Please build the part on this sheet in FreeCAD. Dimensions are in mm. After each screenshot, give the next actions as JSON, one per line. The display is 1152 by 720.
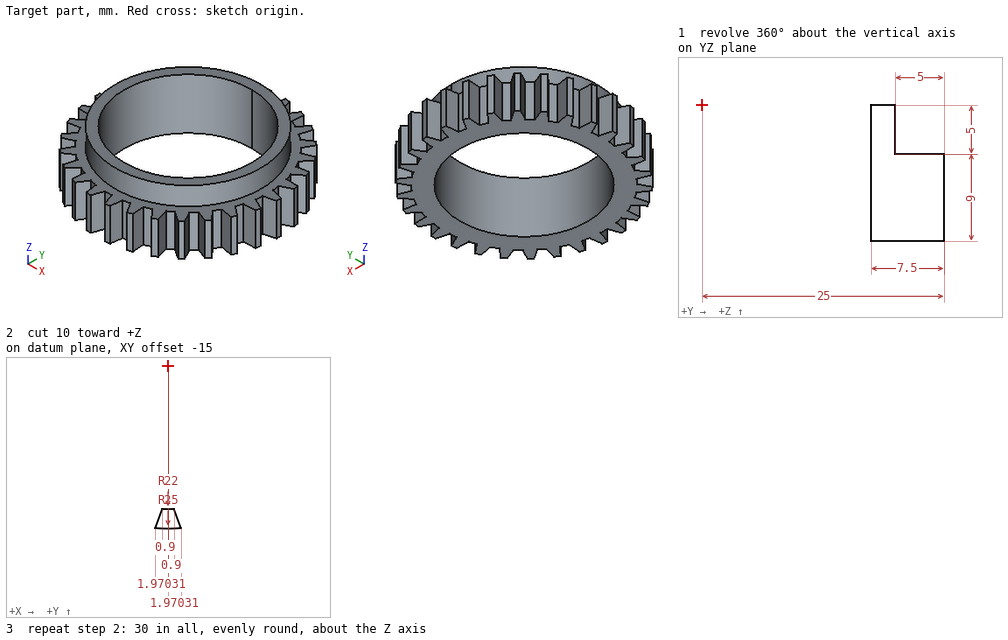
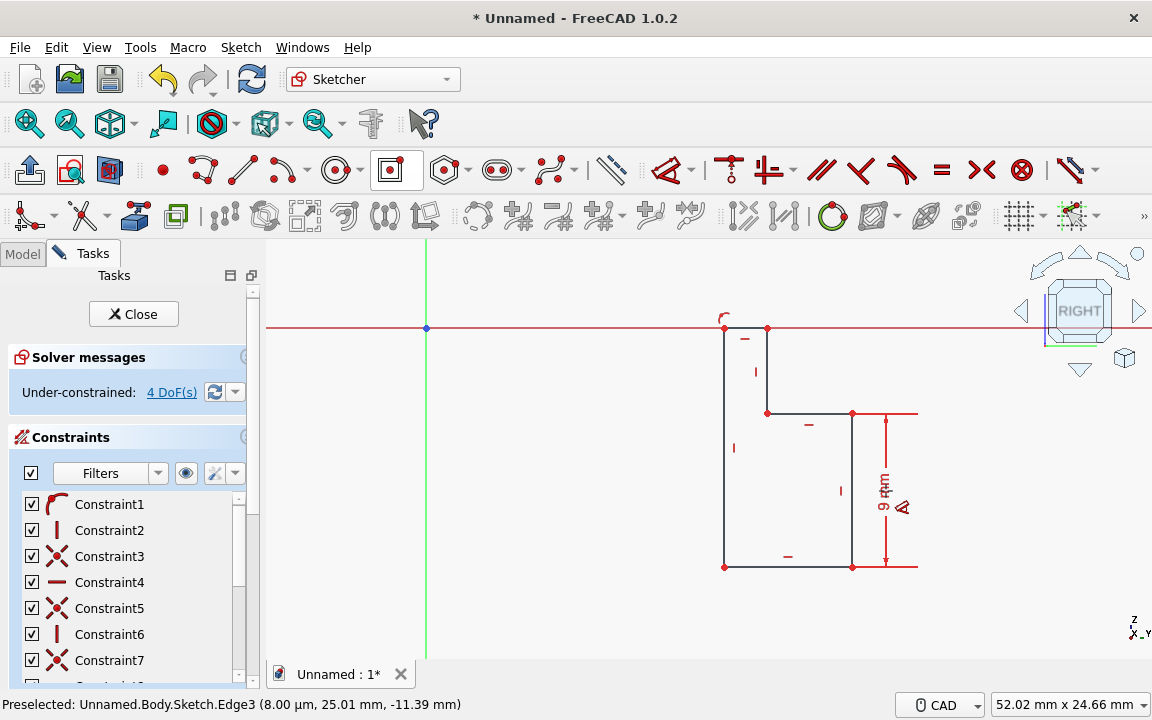
{"action": "left_click", "coordinate": [826, 414]}
{"action": "left_click", "coordinate": [809, 380]}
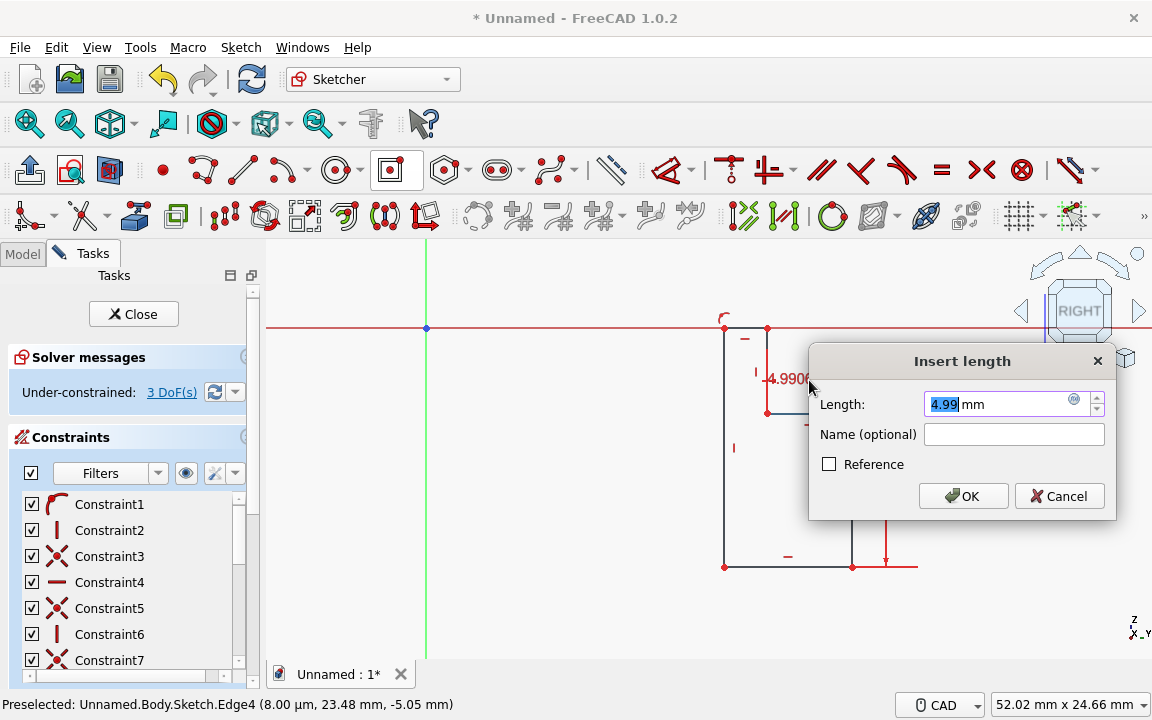
{"action": "type", "text": "5"}
{"action": "key", "text": "Return"}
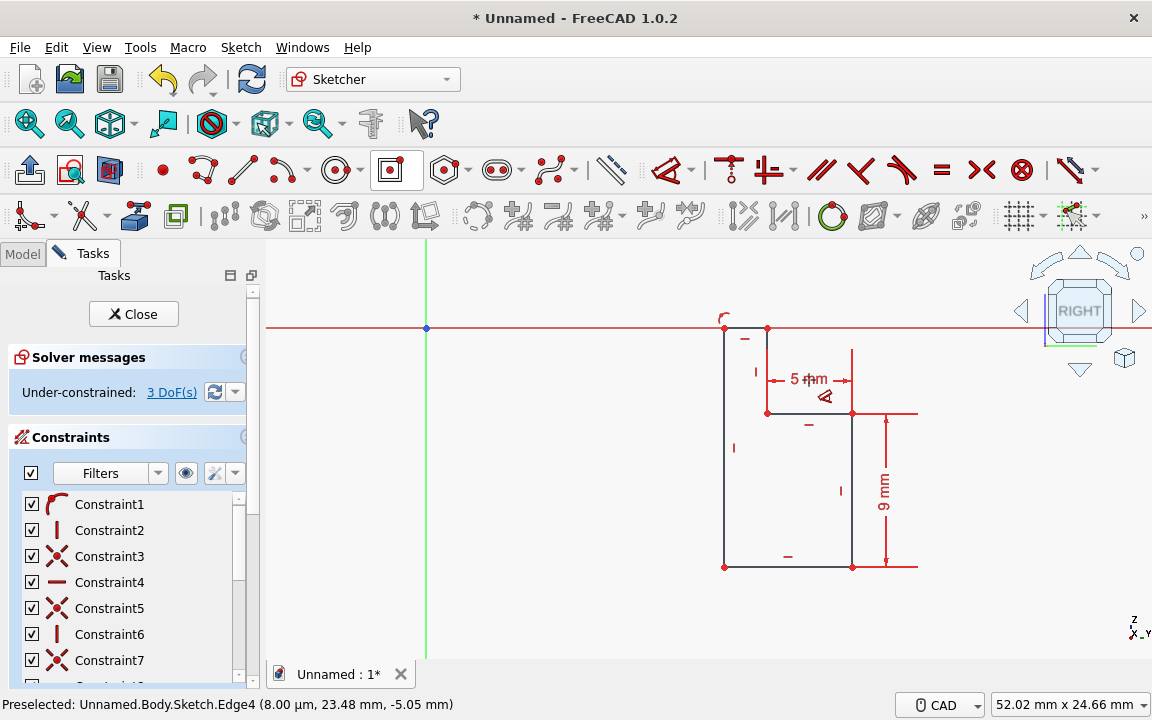
{"action": "left_click", "coordinate": [767, 388]}
{"action": "left_click", "coordinate": [801, 351]}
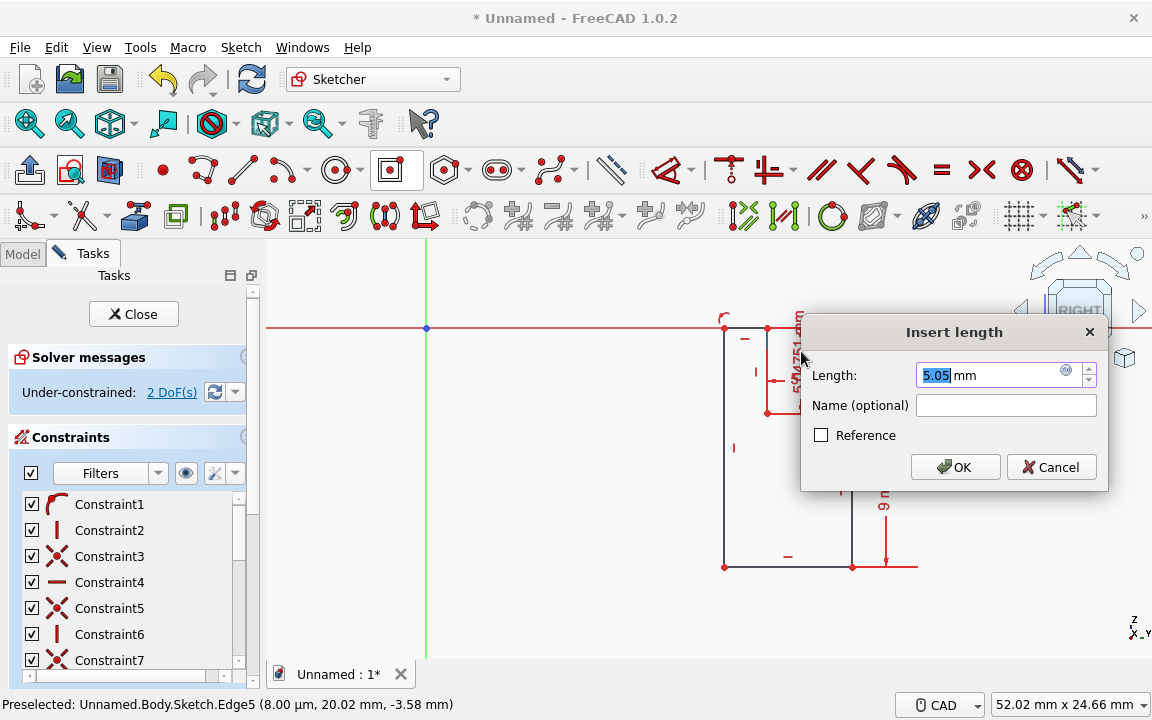
{"action": "type", "text": "5"}
{"action": "key", "text": "Return"}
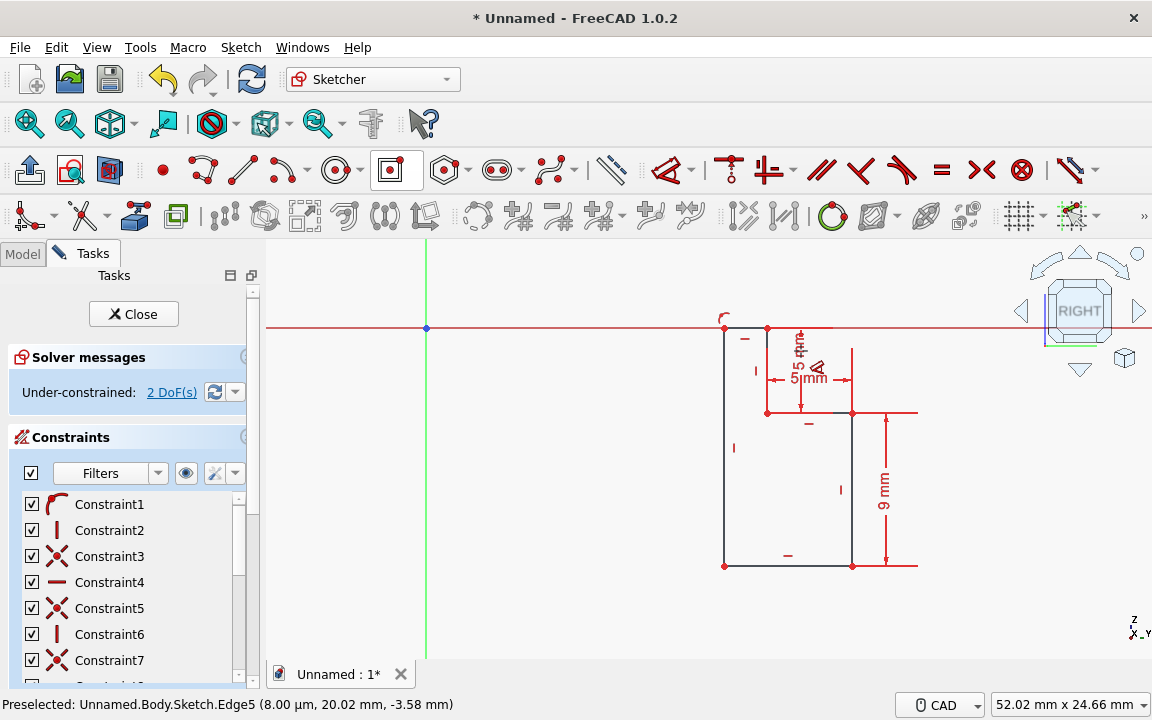
{"action": "left_click", "coordinate": [762, 566]}
{"action": "left_click", "coordinate": [788, 600]}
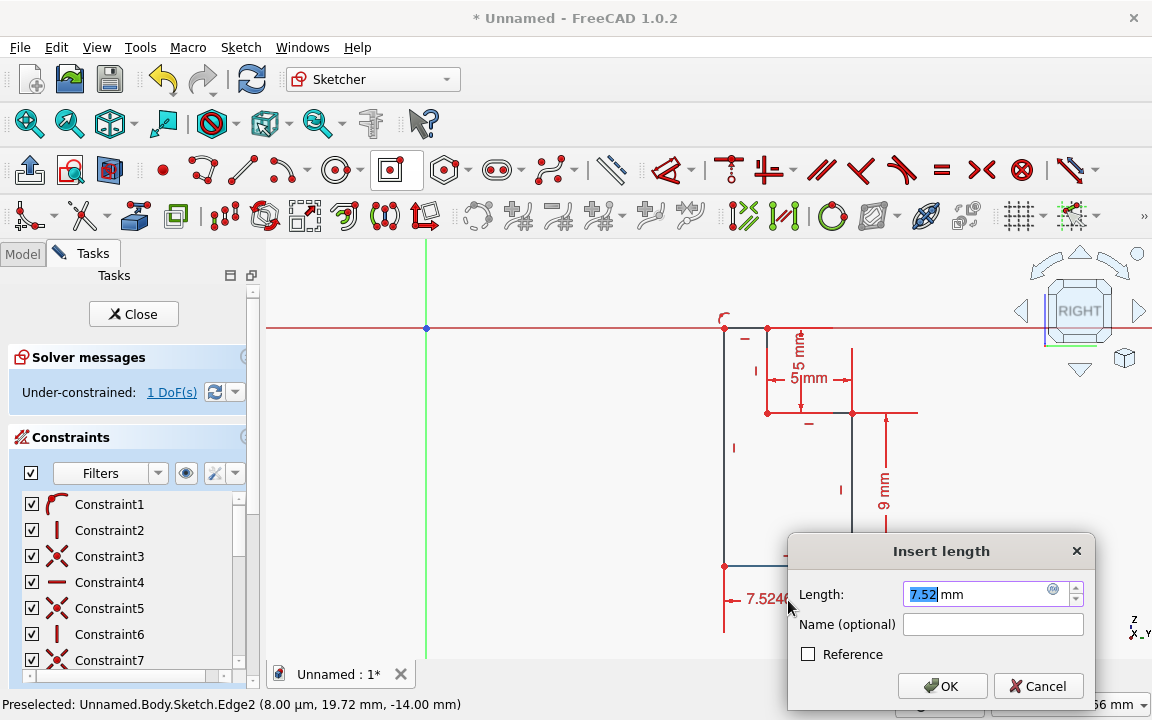
{"action": "type", "text": "7.5"}
{"action": "key", "text": "Return"}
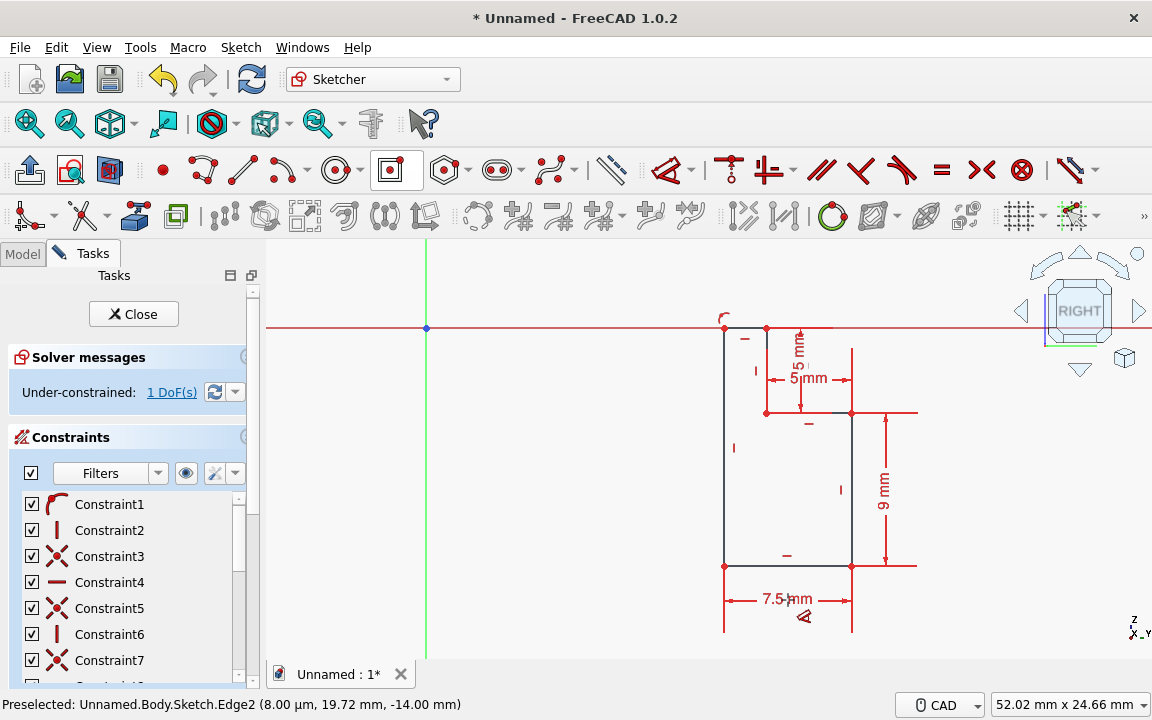
{"action": "left_click", "coordinate": [852, 566]}
{"action": "left_click", "coordinate": [639, 600]}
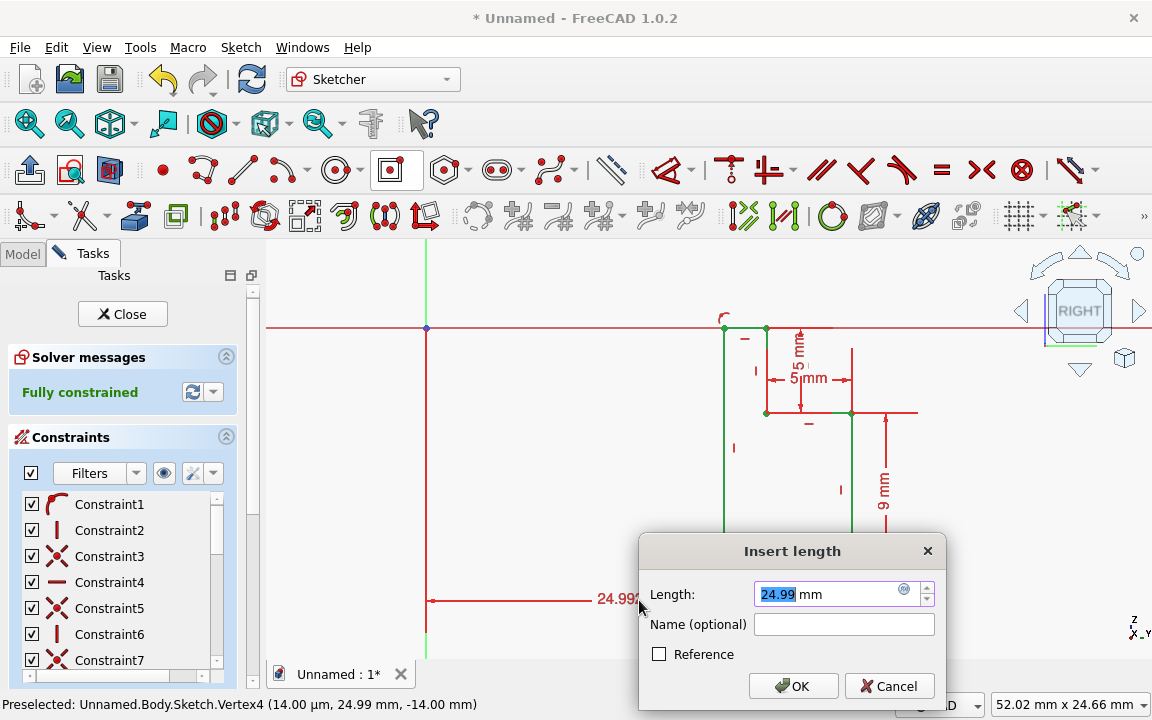
{"action": "type", "text": "25"}
{"action": "key", "text": "Return"}
{"action": "key", "text": "Escape"}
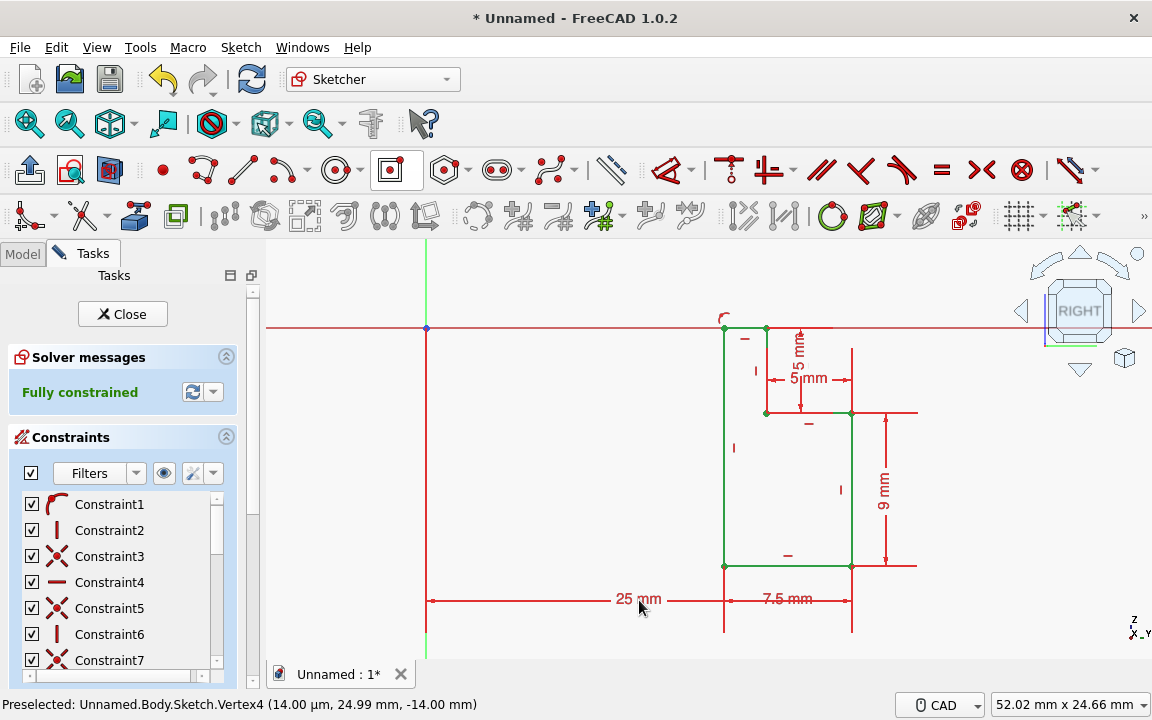
{"action": "left_click", "coordinate": [123, 314]}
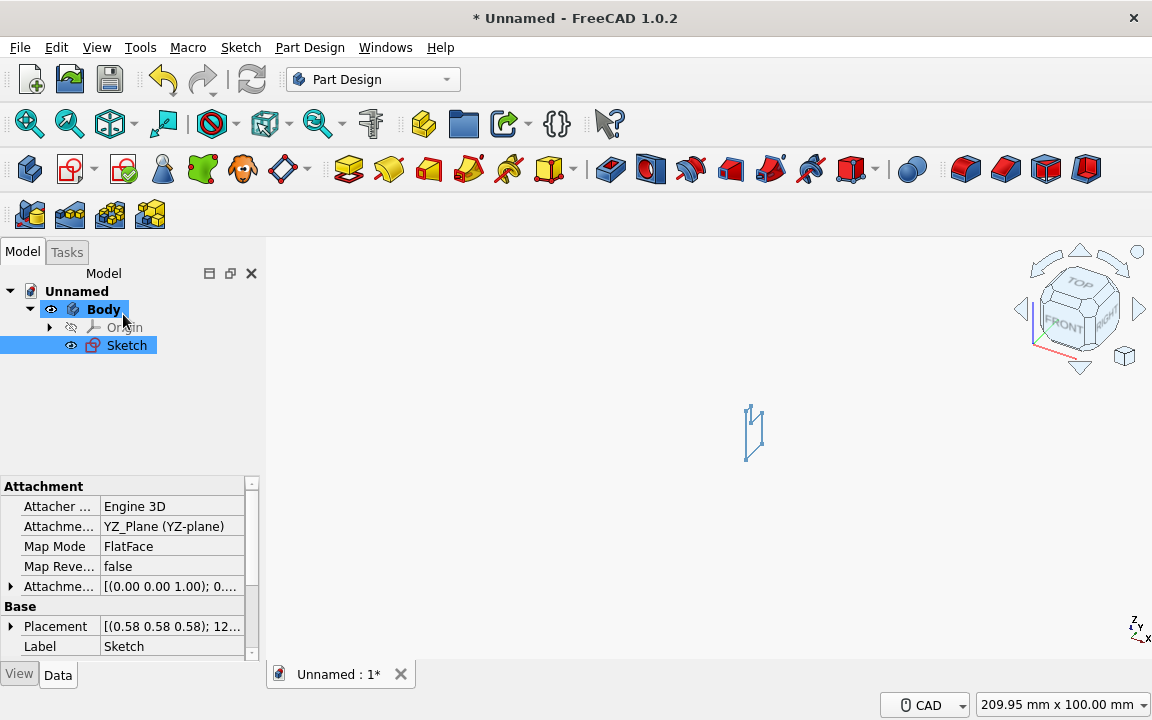
{"action": "left_click", "coordinate": [390, 170]}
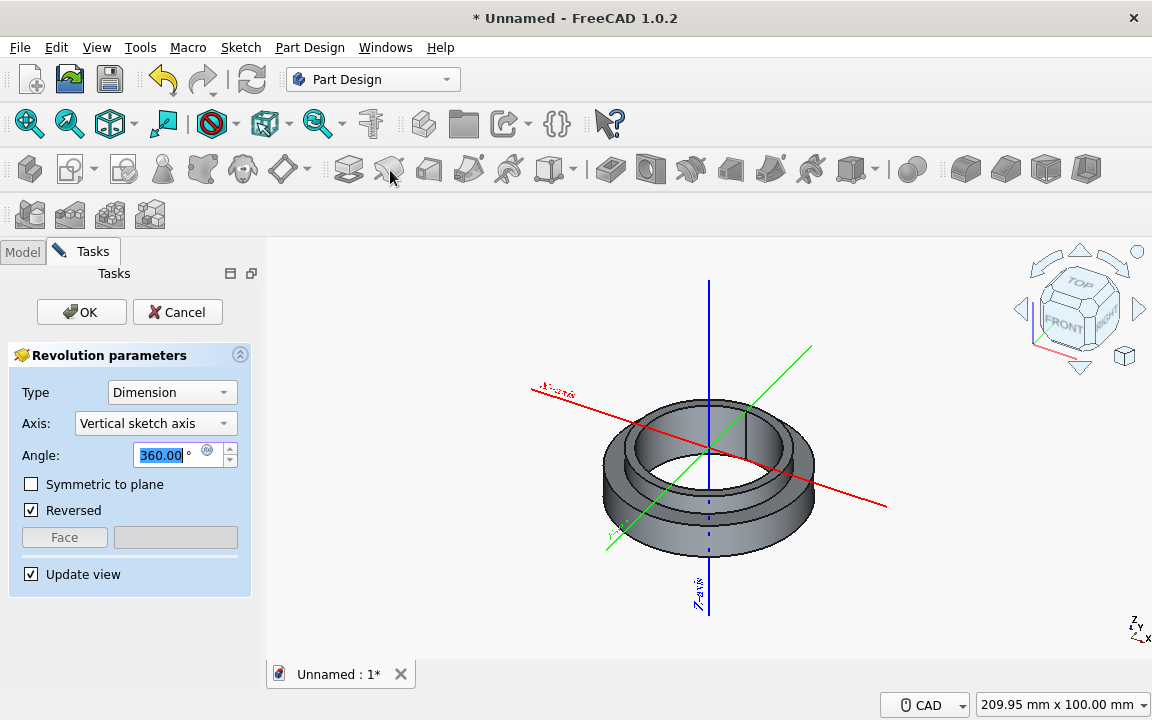
{"action": "left_click", "coordinate": [82, 312]}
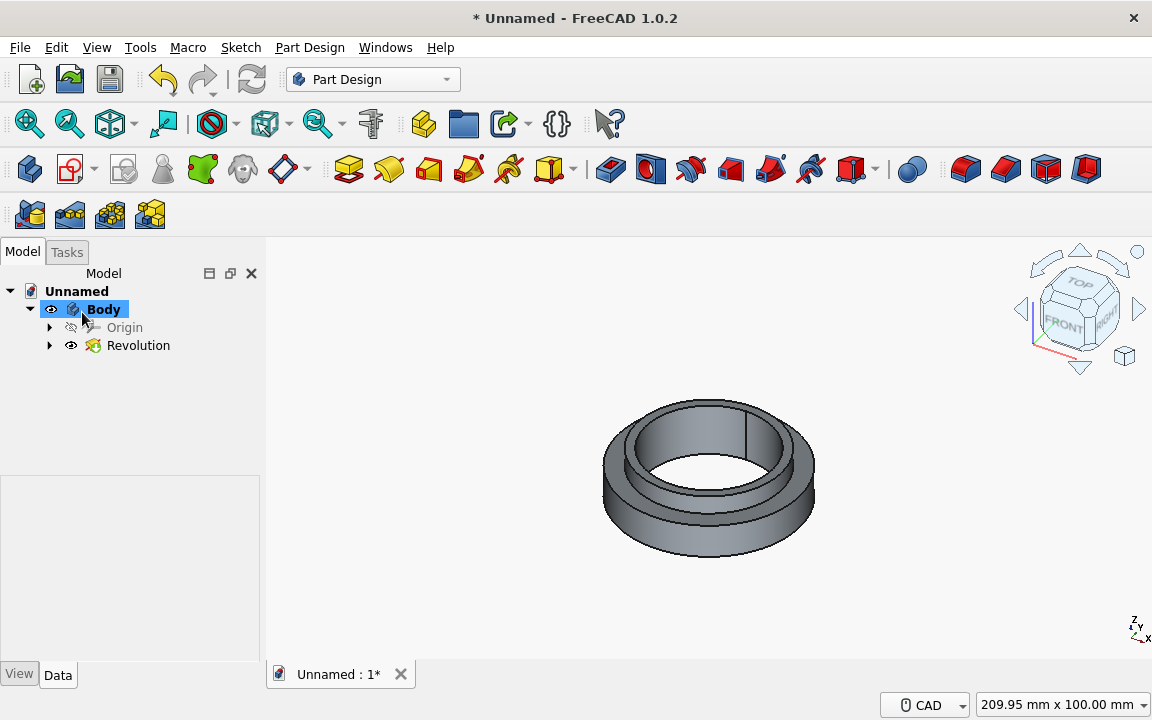
{"action": "left_click", "coordinate": [50, 327]}